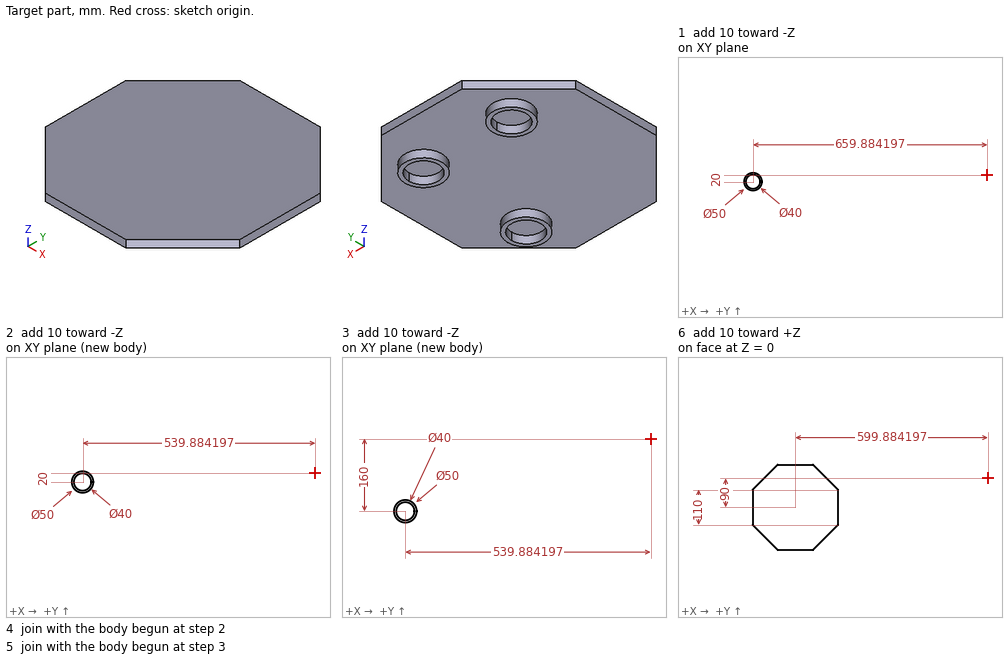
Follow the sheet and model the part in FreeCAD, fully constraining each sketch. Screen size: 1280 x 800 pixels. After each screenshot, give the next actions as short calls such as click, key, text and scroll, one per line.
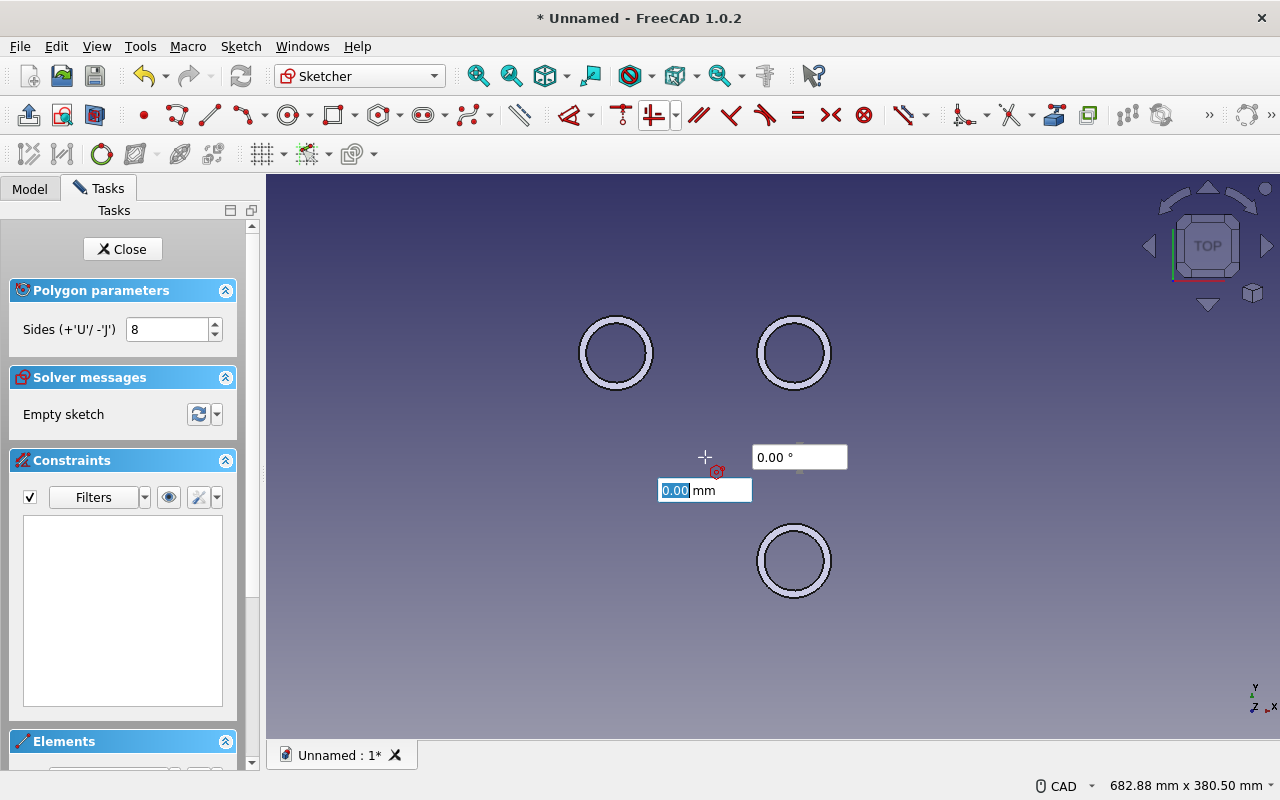
click(787, 654)
right_click(787, 654)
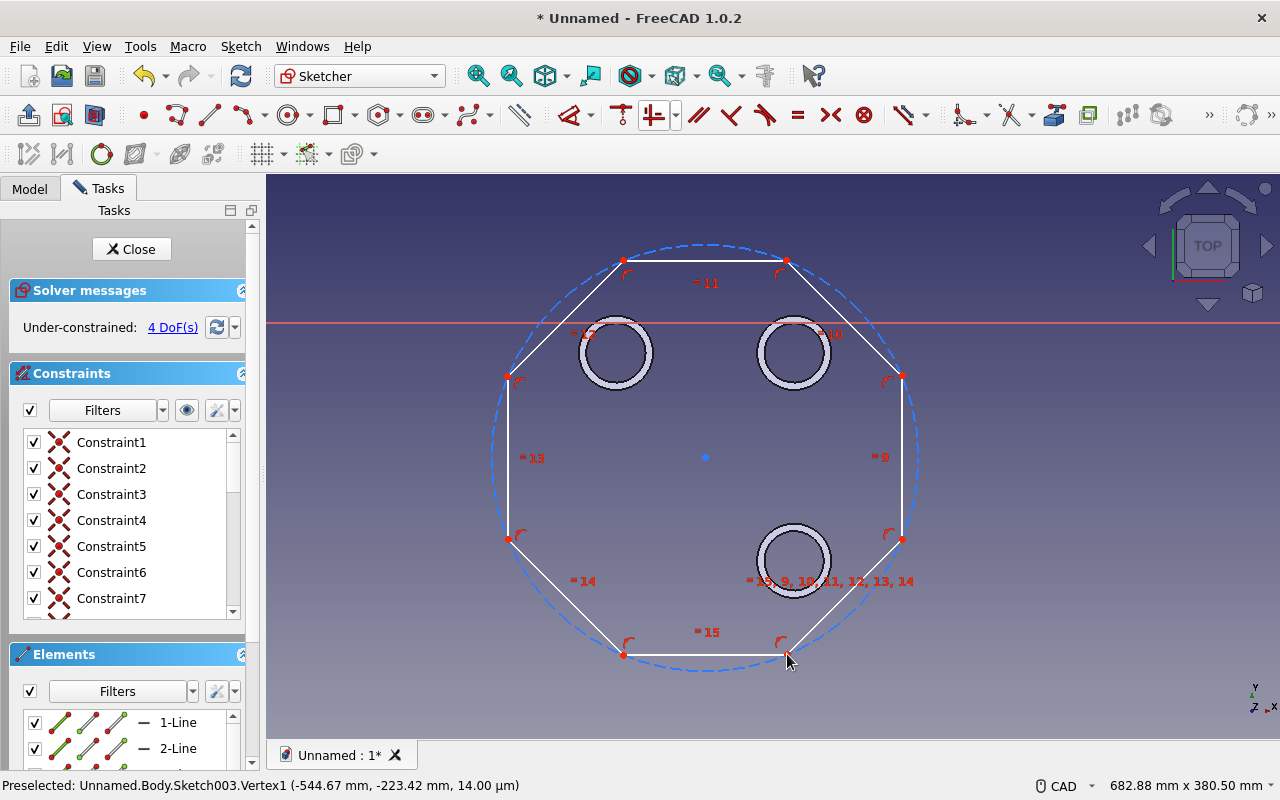
click(902, 490)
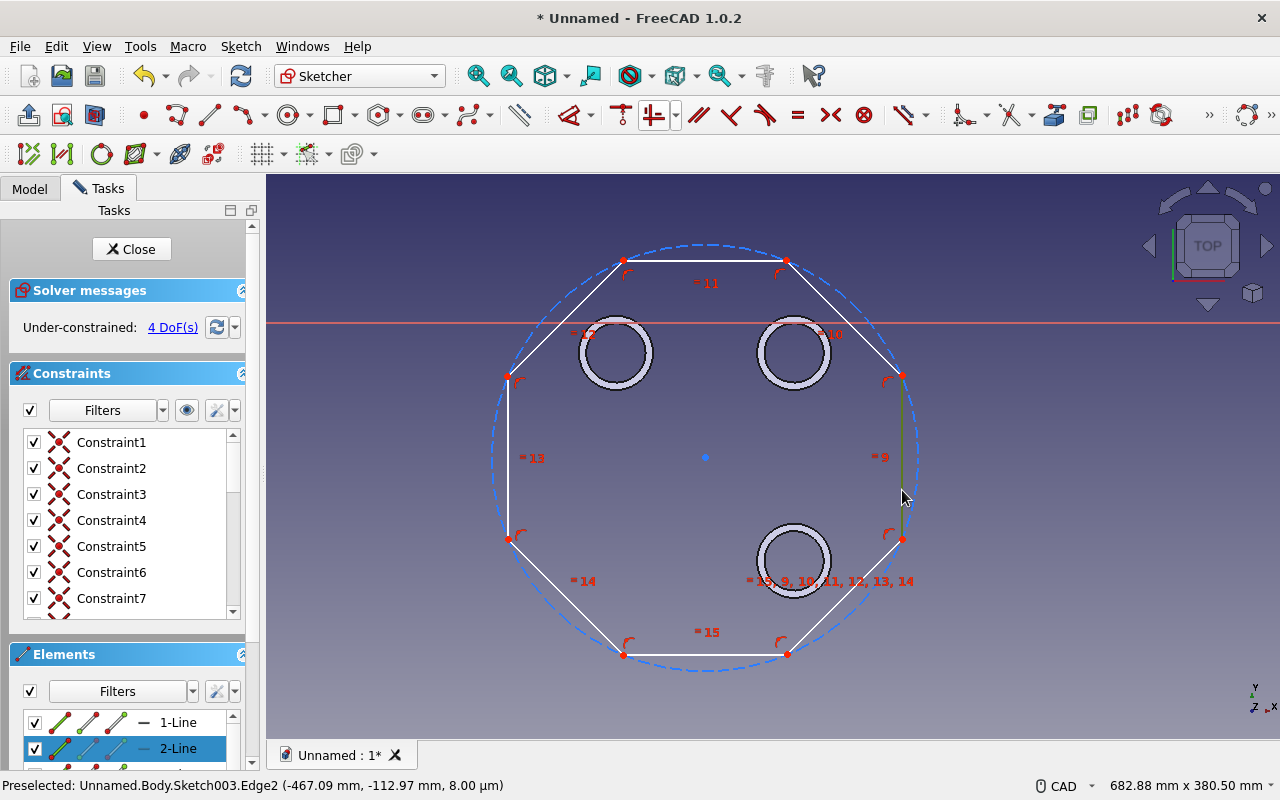
key(v)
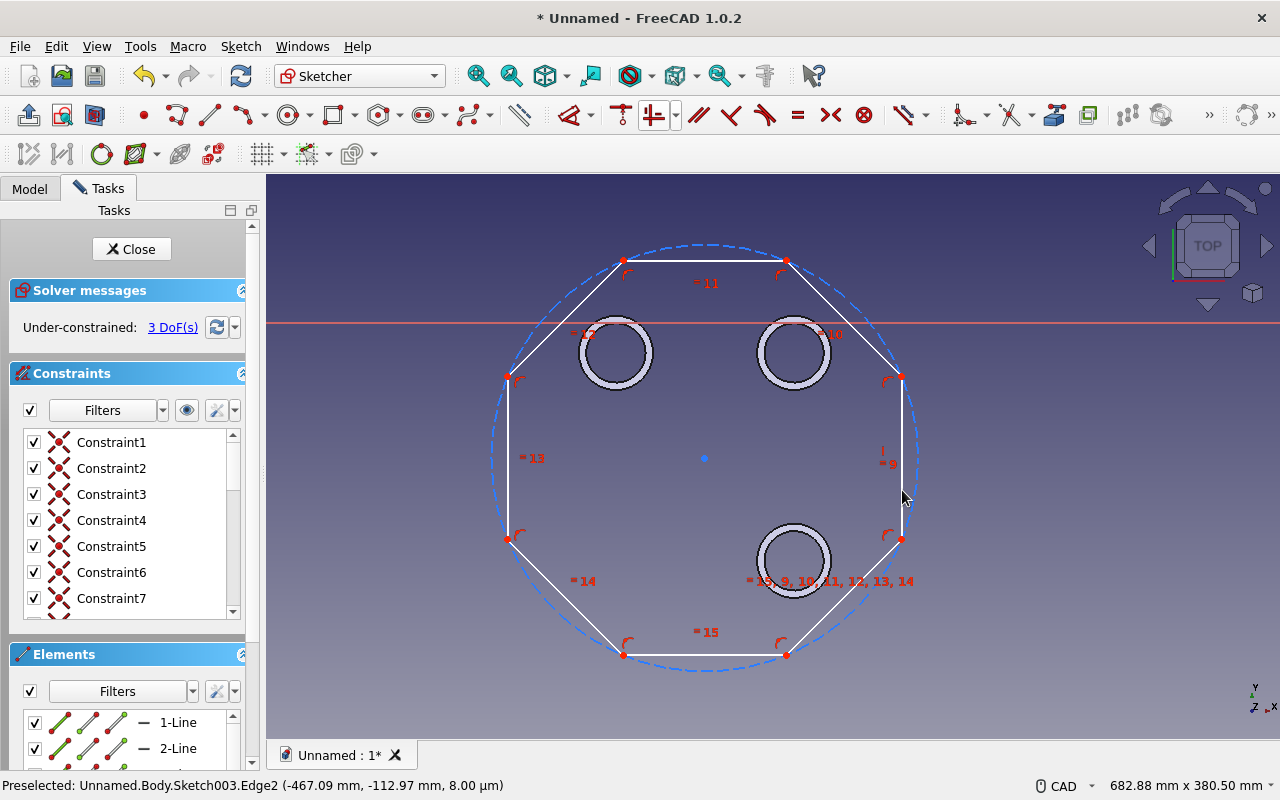
key(d)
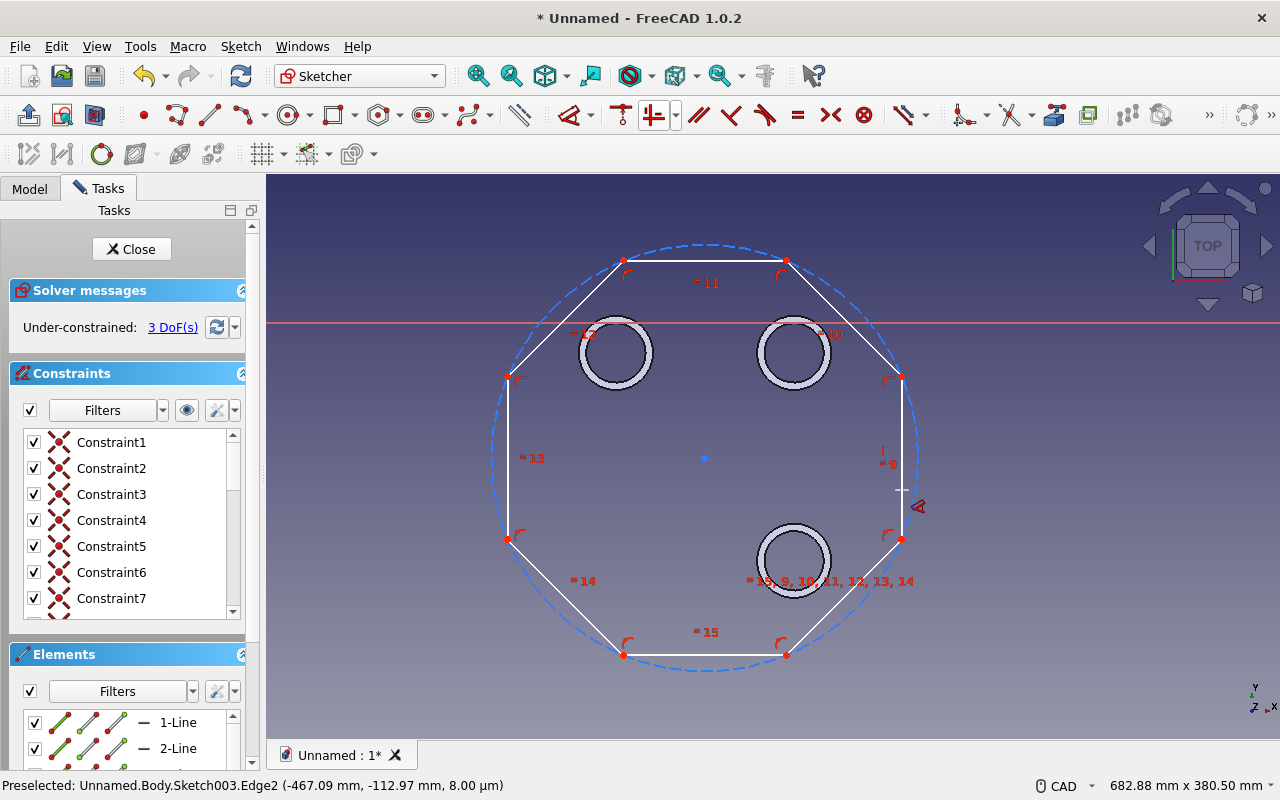
click(705, 458)
click(671, 391)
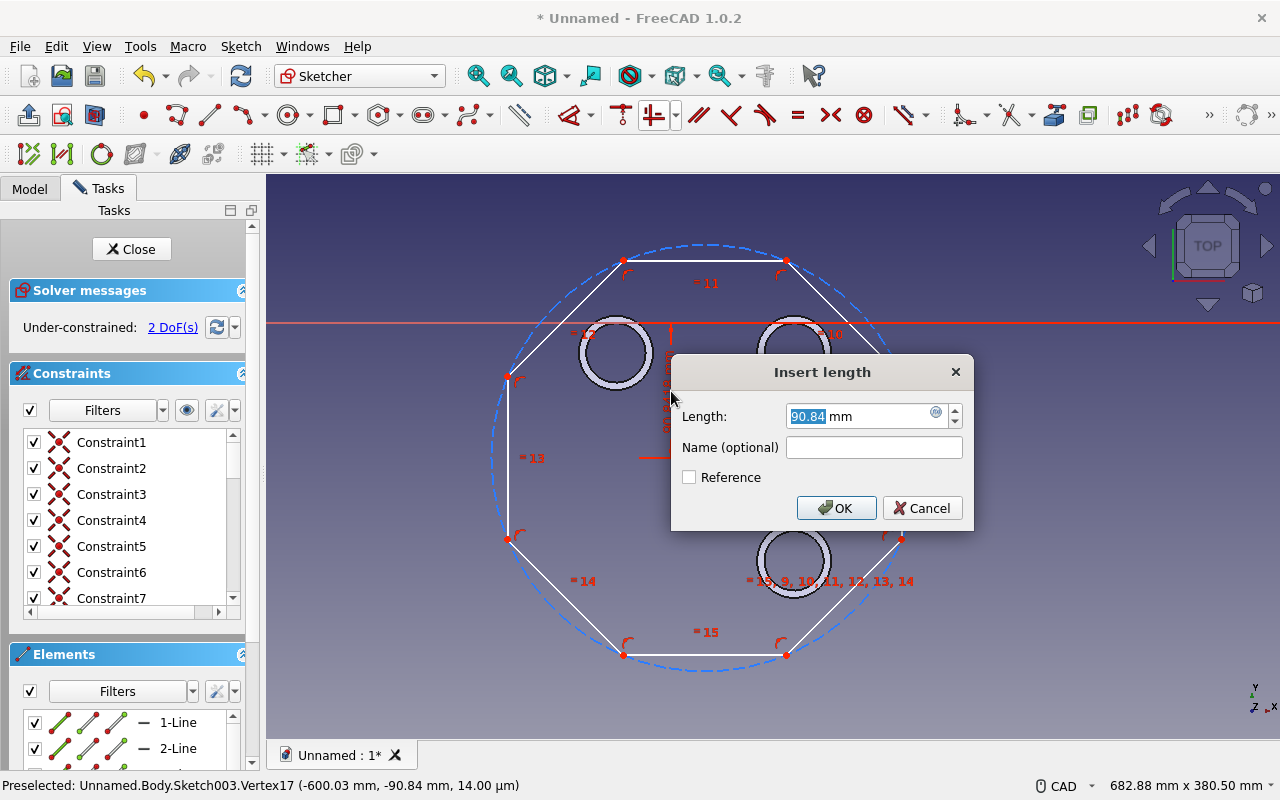
text(90)
key(Return)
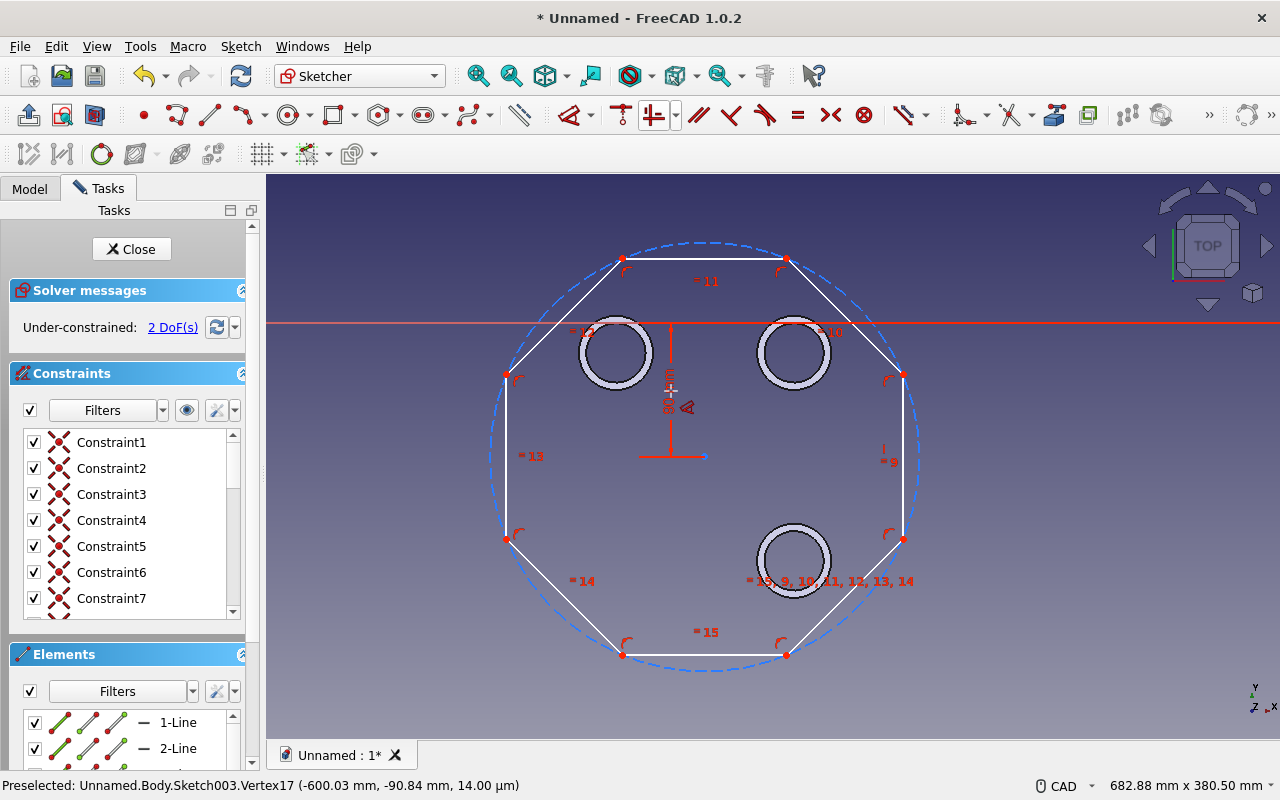
click(903, 490)
click(937, 457)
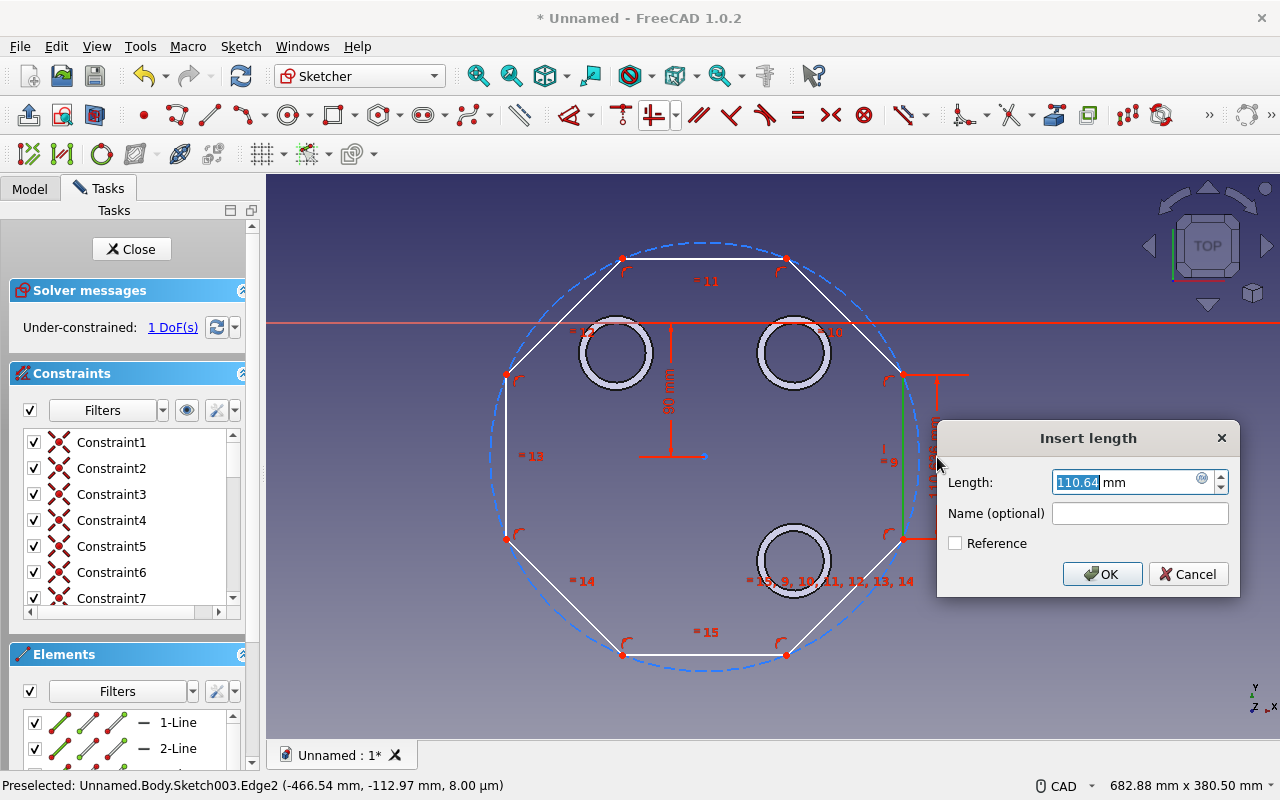
text(110)
key(Return)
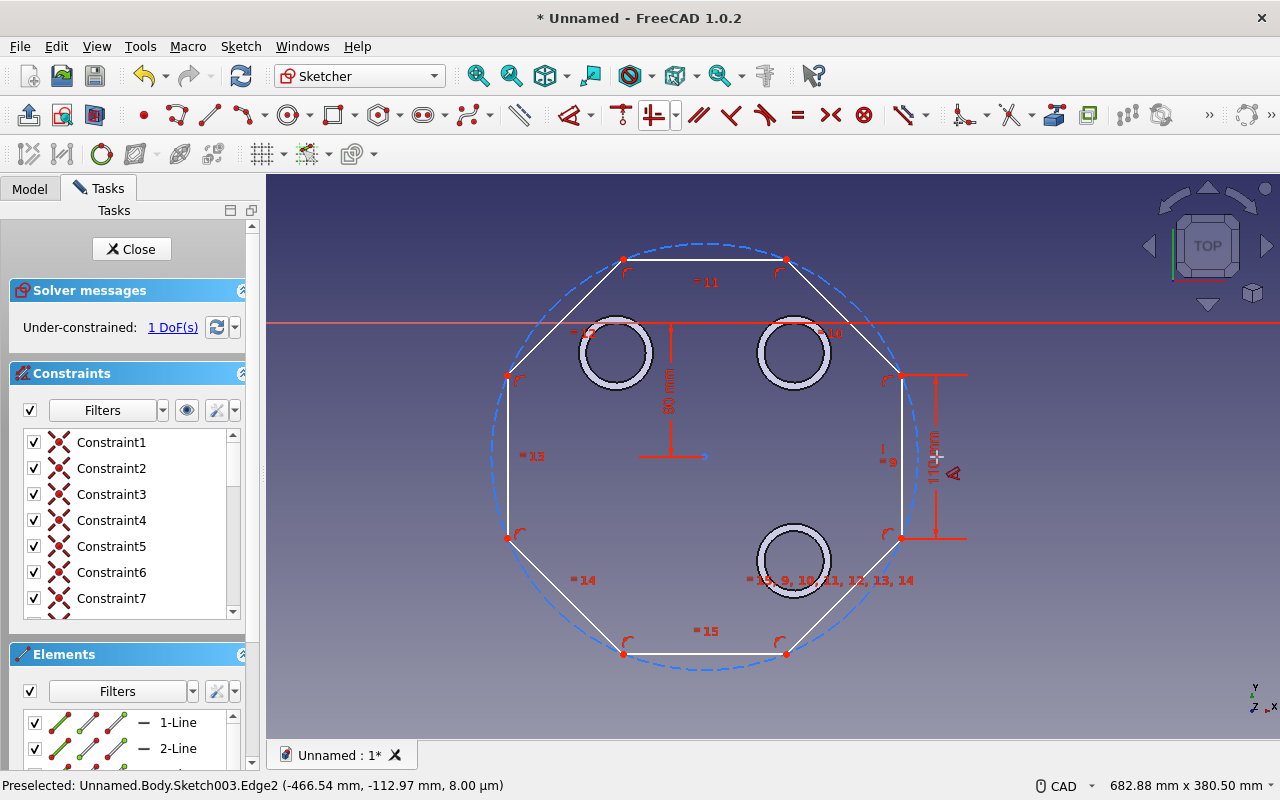
click(705, 457)
click(910, 289)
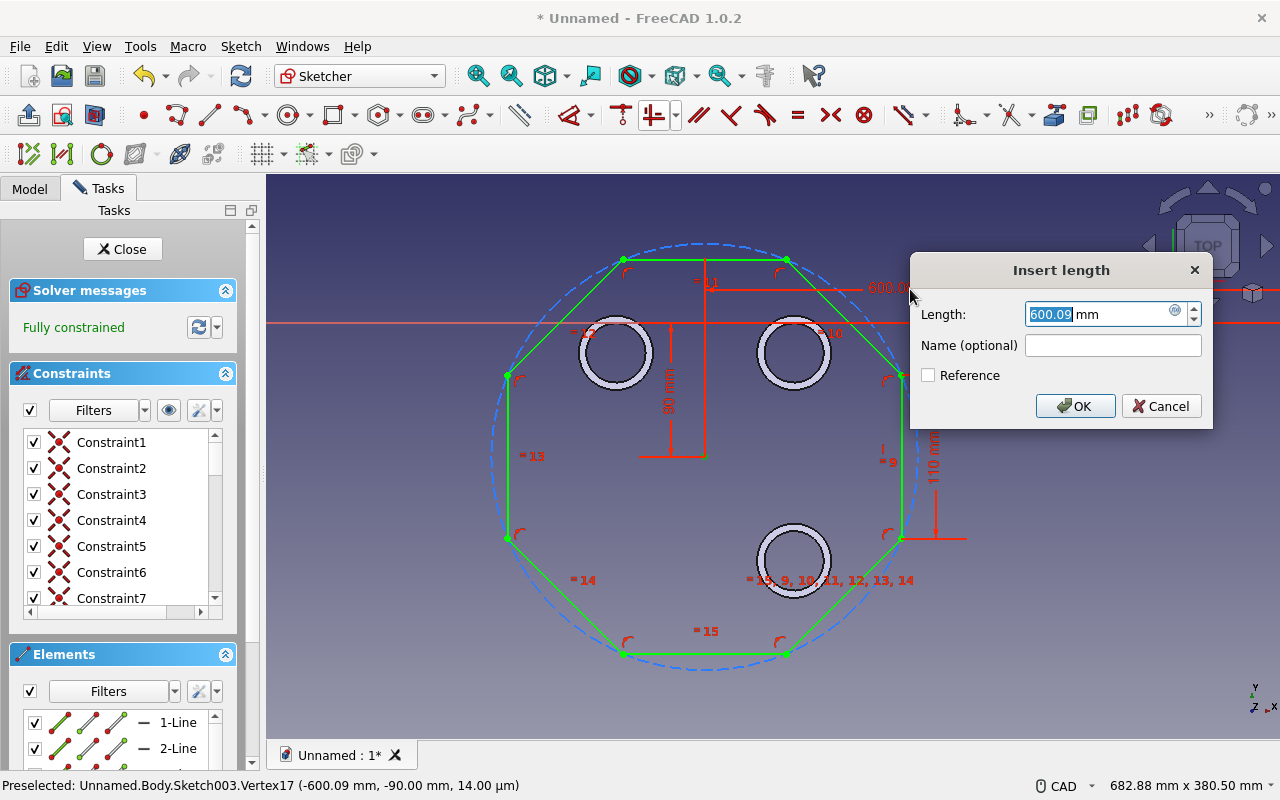
text(599.884197)
key(Return)
key(Escape)